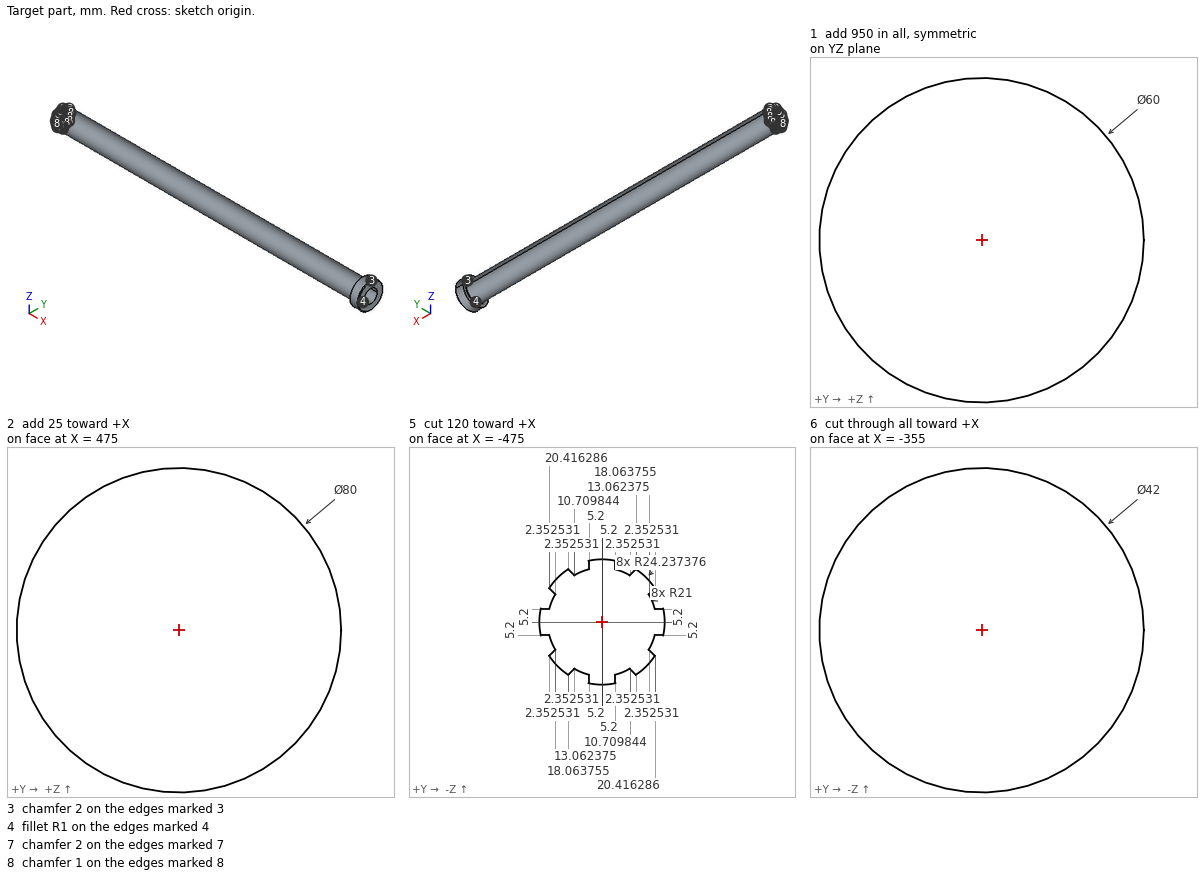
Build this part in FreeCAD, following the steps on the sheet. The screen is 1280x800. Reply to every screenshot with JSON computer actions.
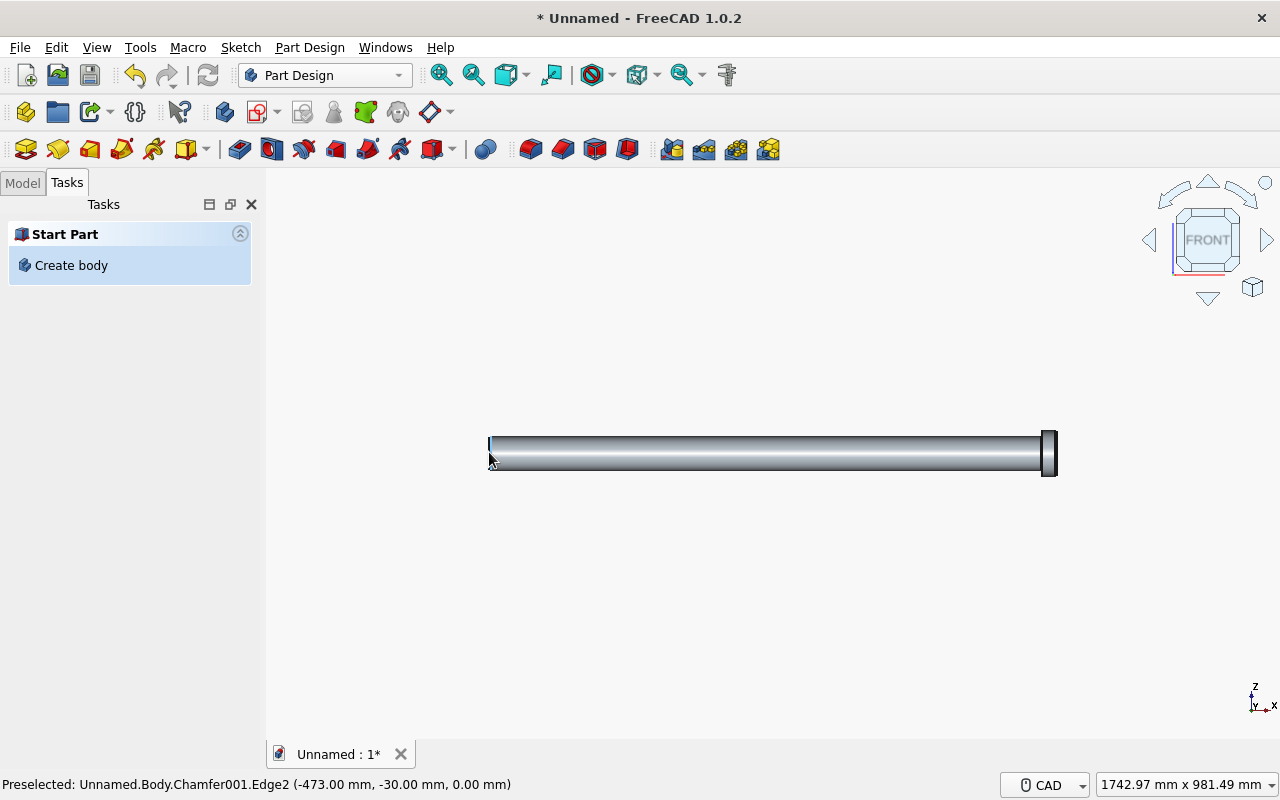
{"action": "key", "text": "3"}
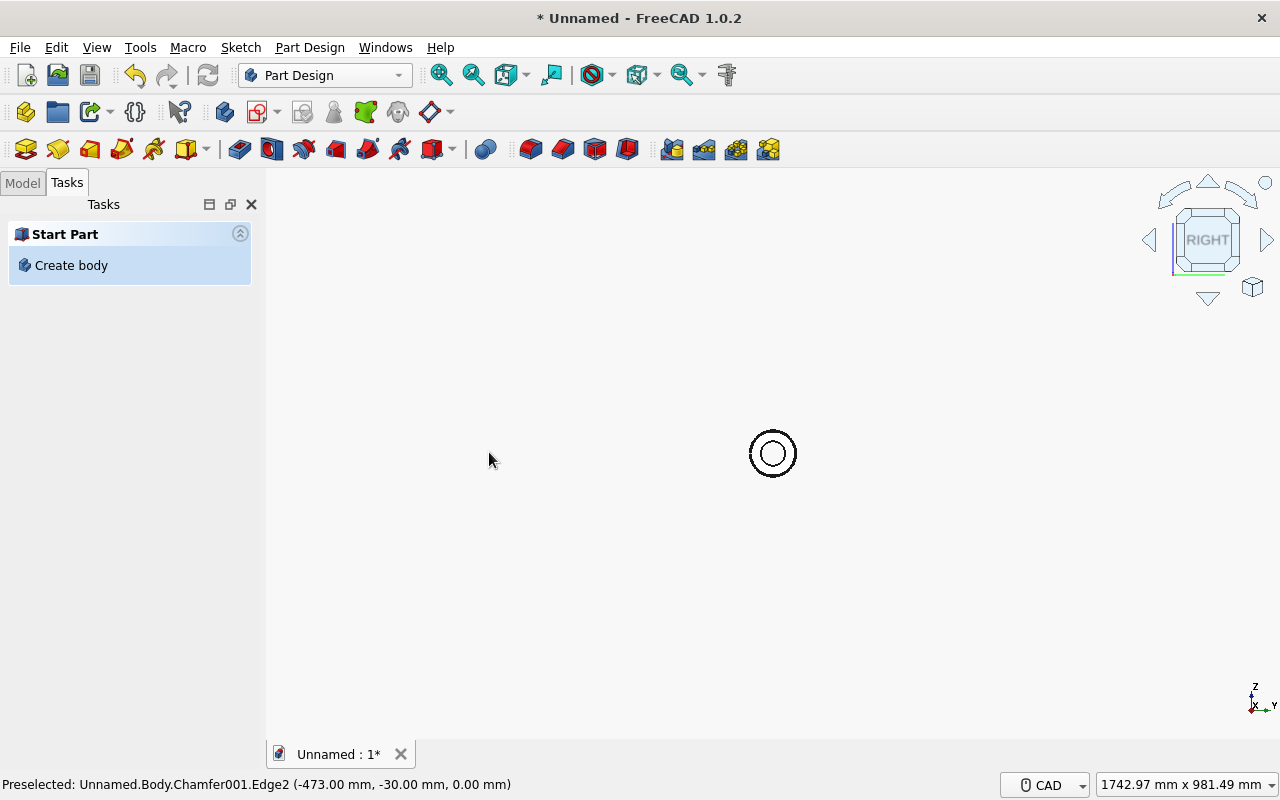
{"action": "key", "text": "v f"}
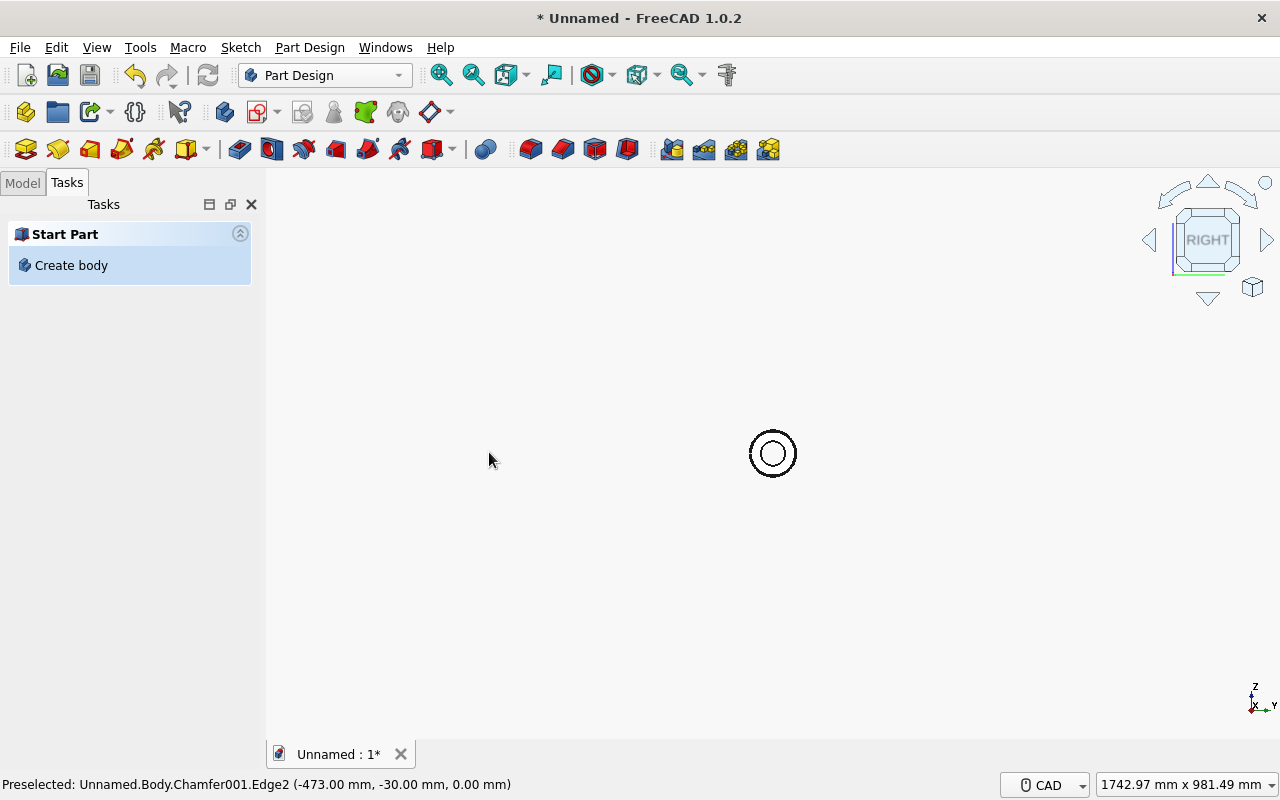
{"action": "scroll", "coordinate": [759, 452], "scroll_direction": "up", "scroll_amount": 10}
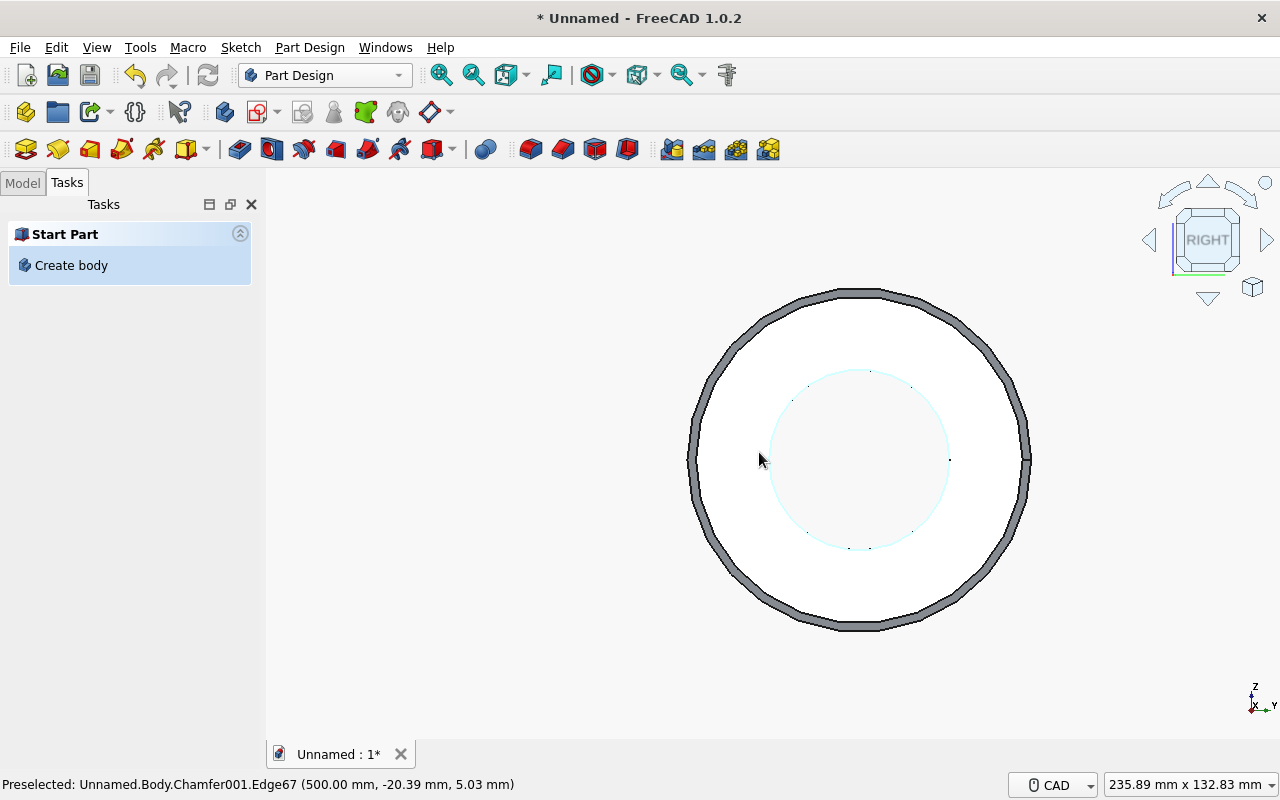
{"action": "left_click", "coordinate": [442, 76]}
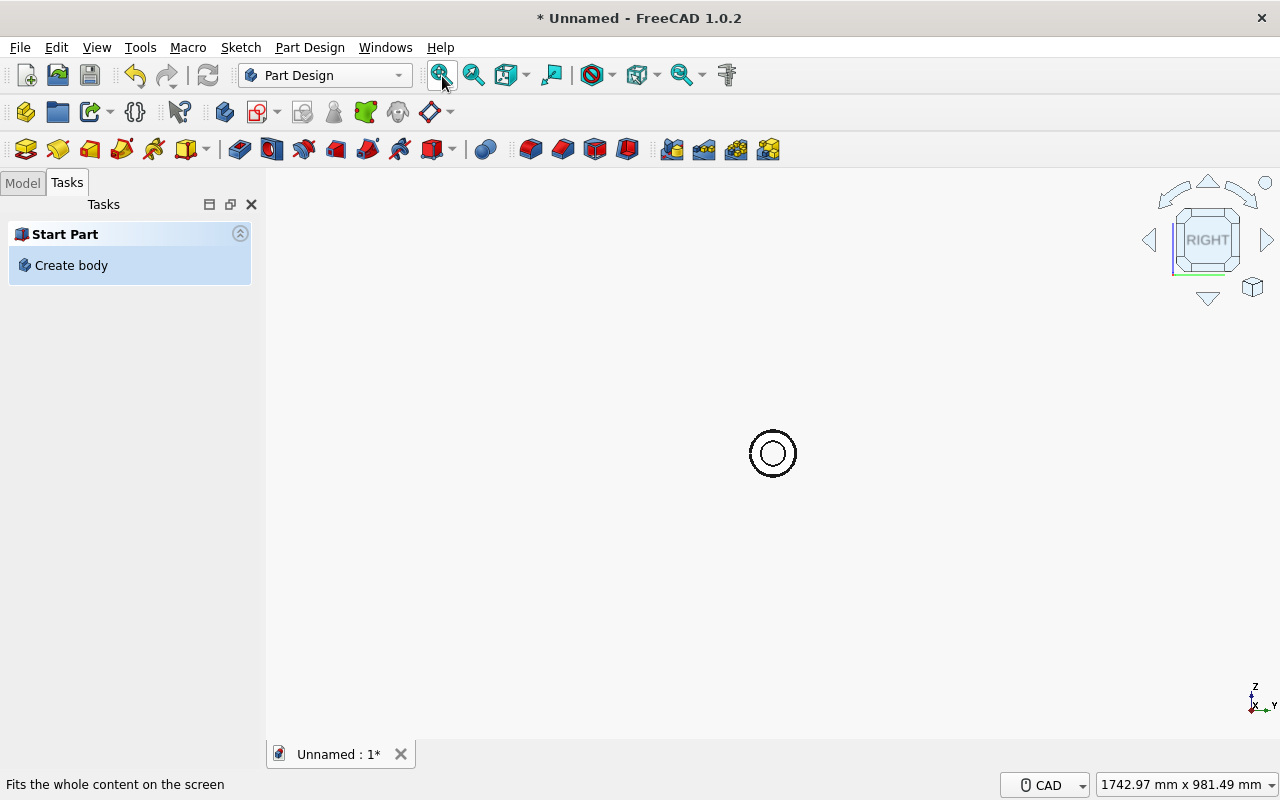
{"action": "key", "text": "5"}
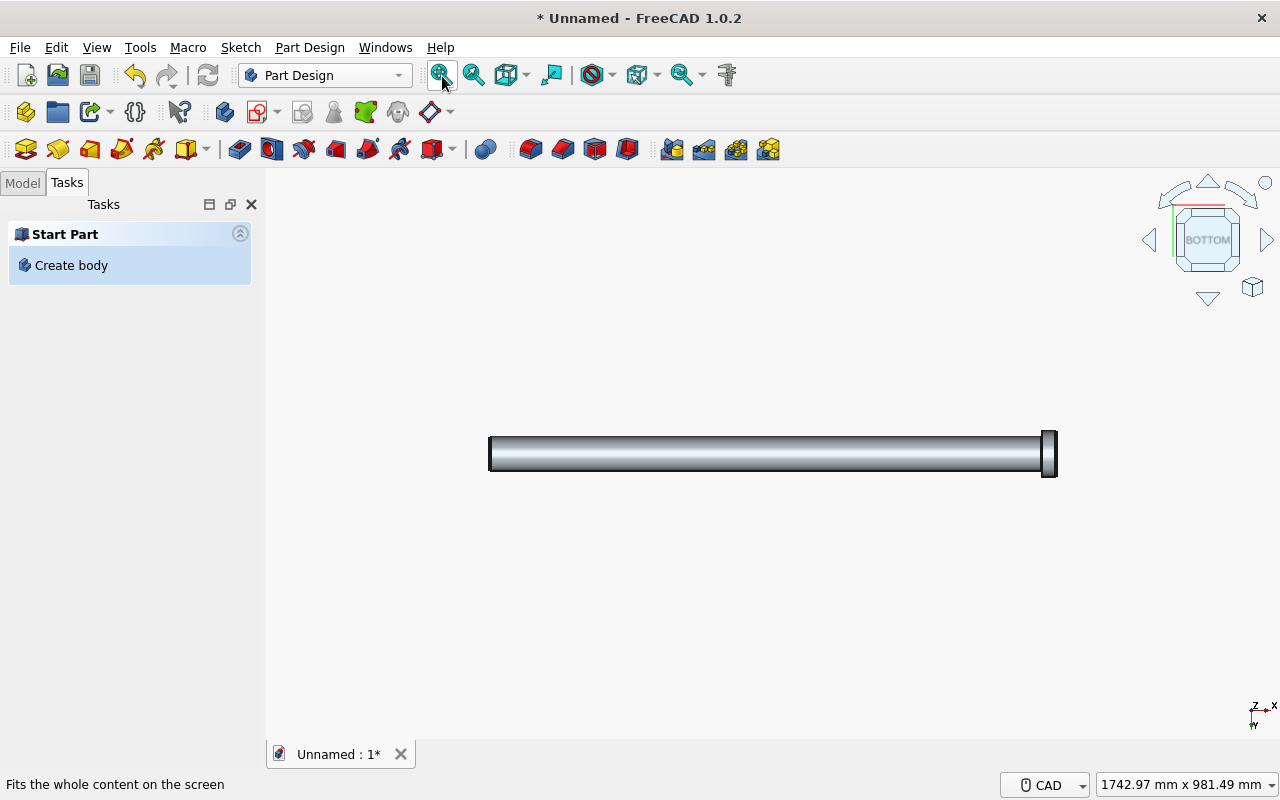
{"action": "scroll", "coordinate": [489, 438], "scroll_direction": "up", "scroll_amount": 10}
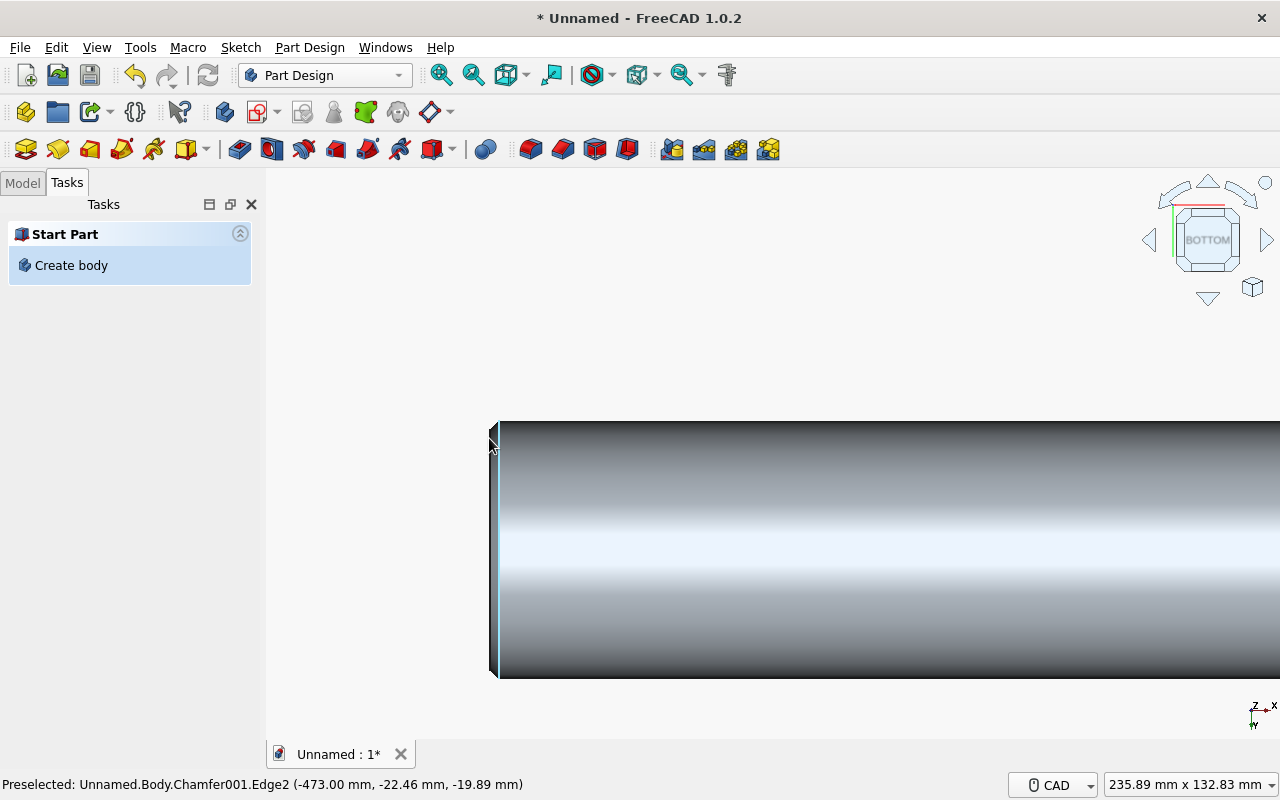
{"action": "key", "text": "v f"}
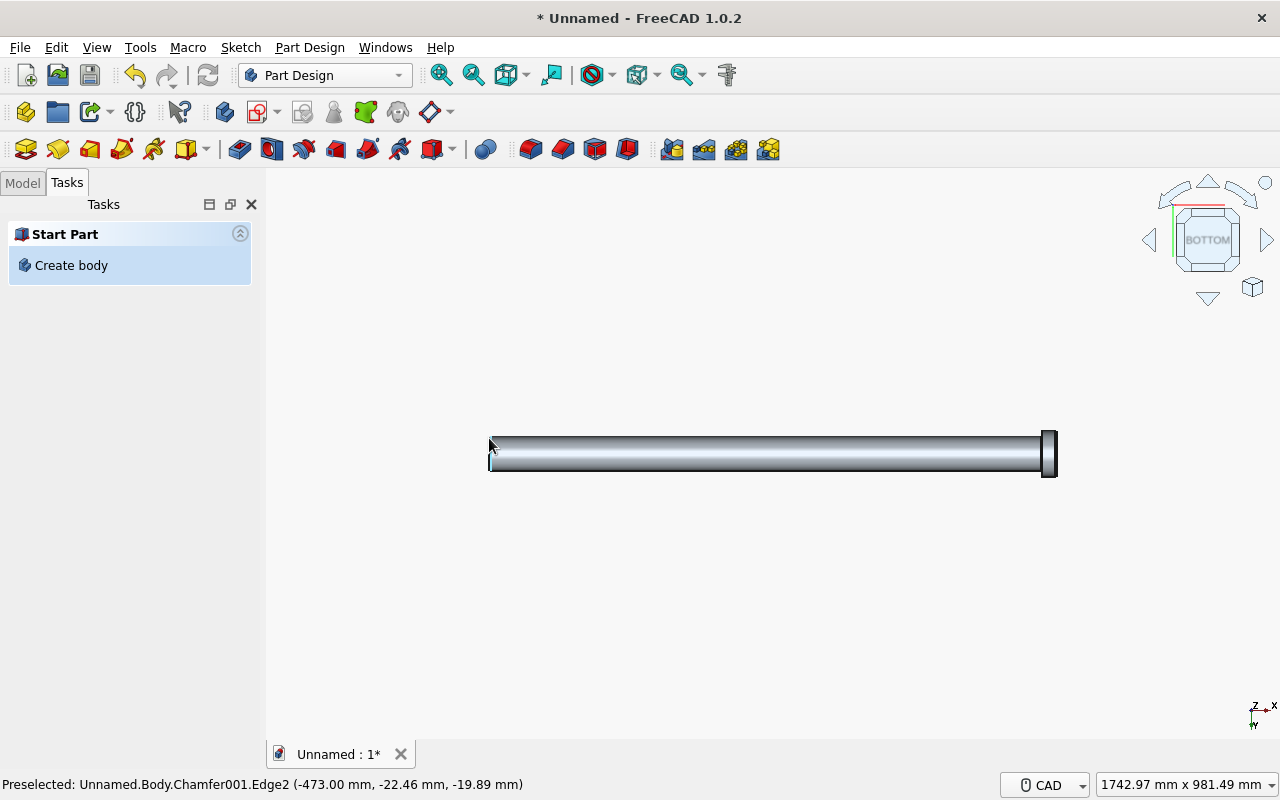
{"action": "key", "text": "4"}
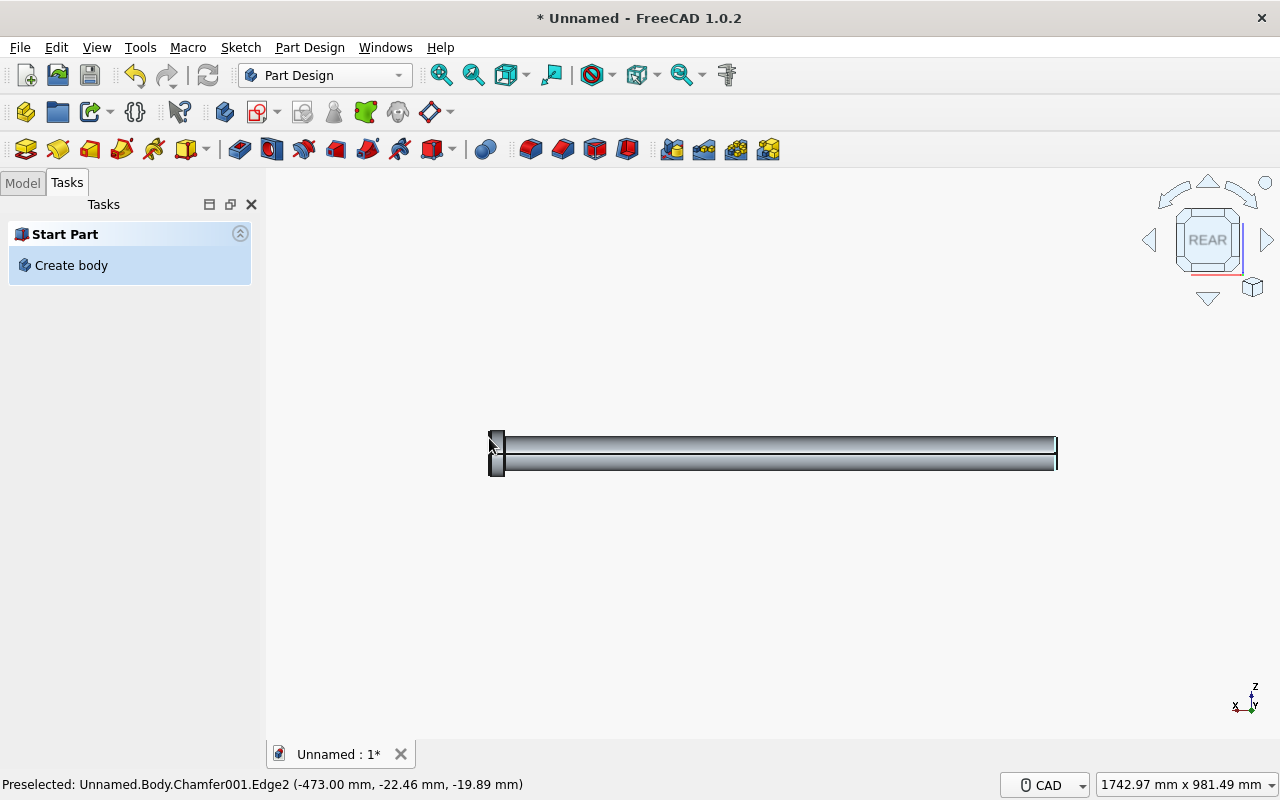
{"action": "scroll", "coordinate": [1057, 452], "scroll_direction": "up", "scroll_amount": 10}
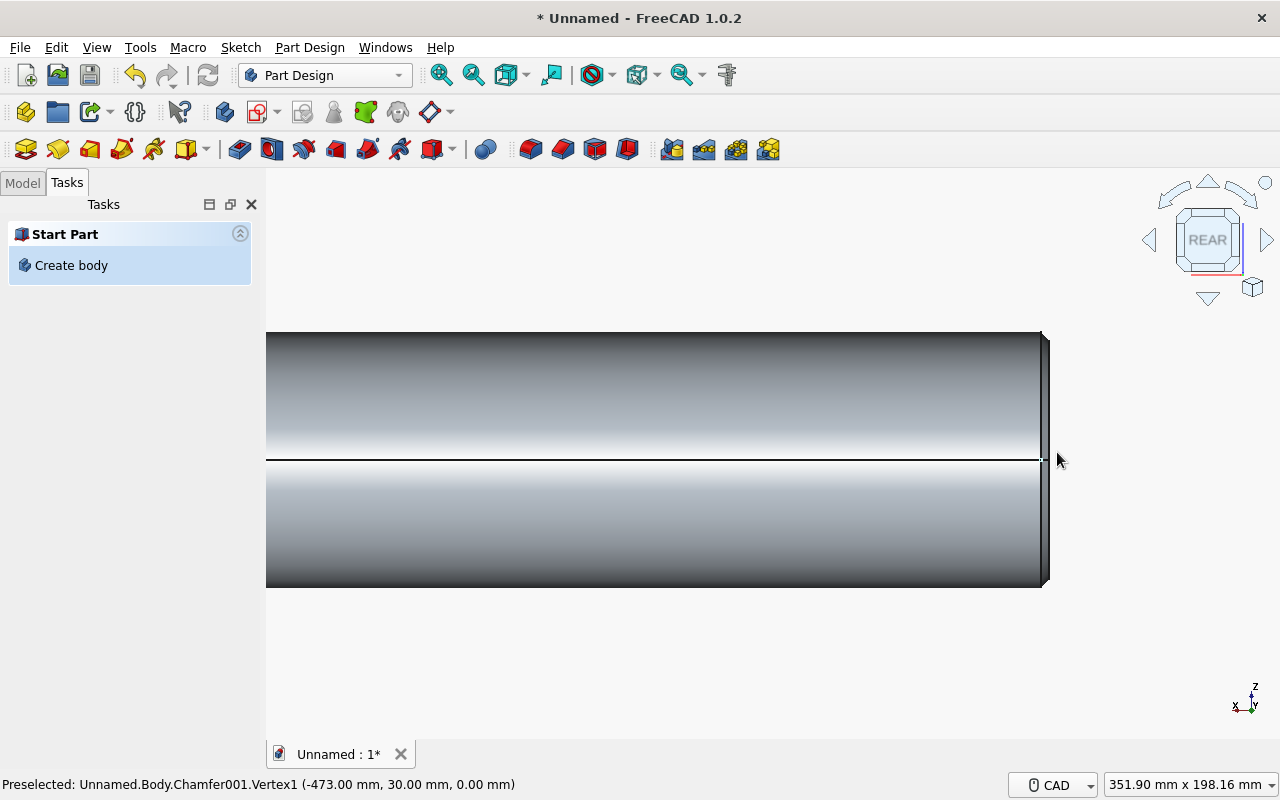
{"action": "key", "text": "v f"}